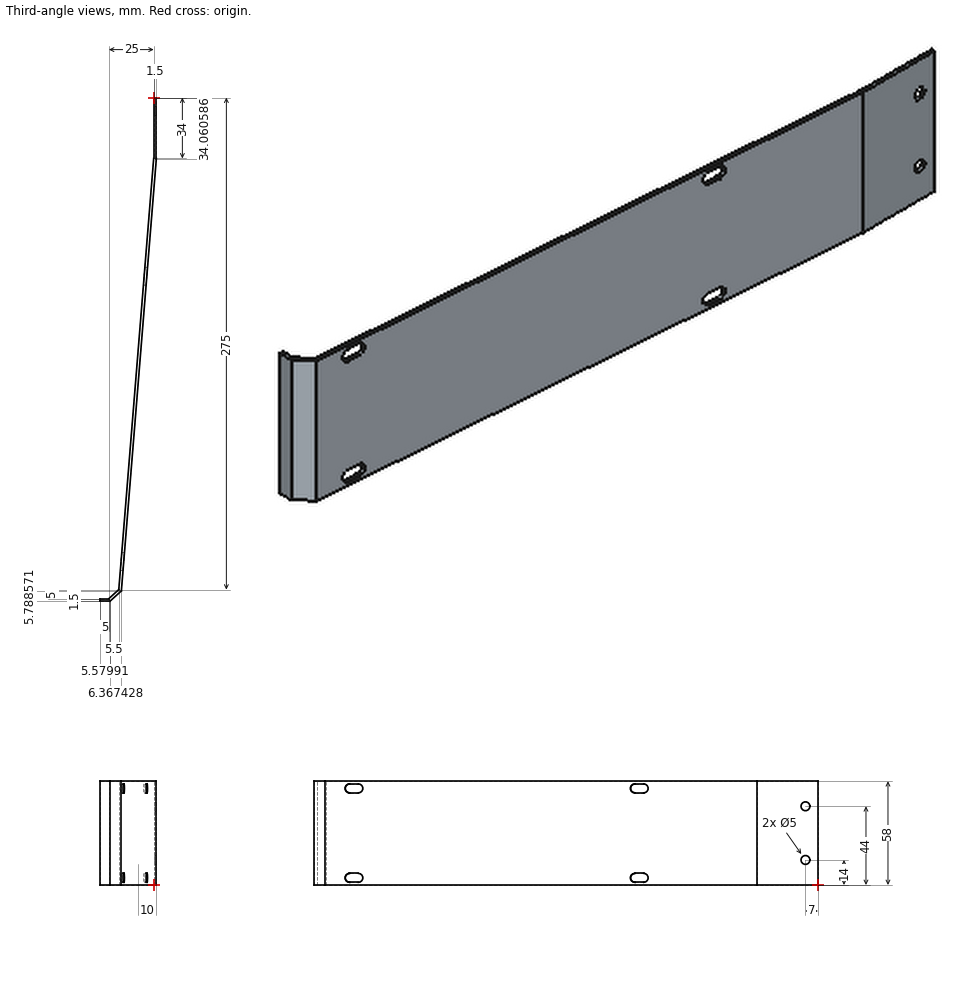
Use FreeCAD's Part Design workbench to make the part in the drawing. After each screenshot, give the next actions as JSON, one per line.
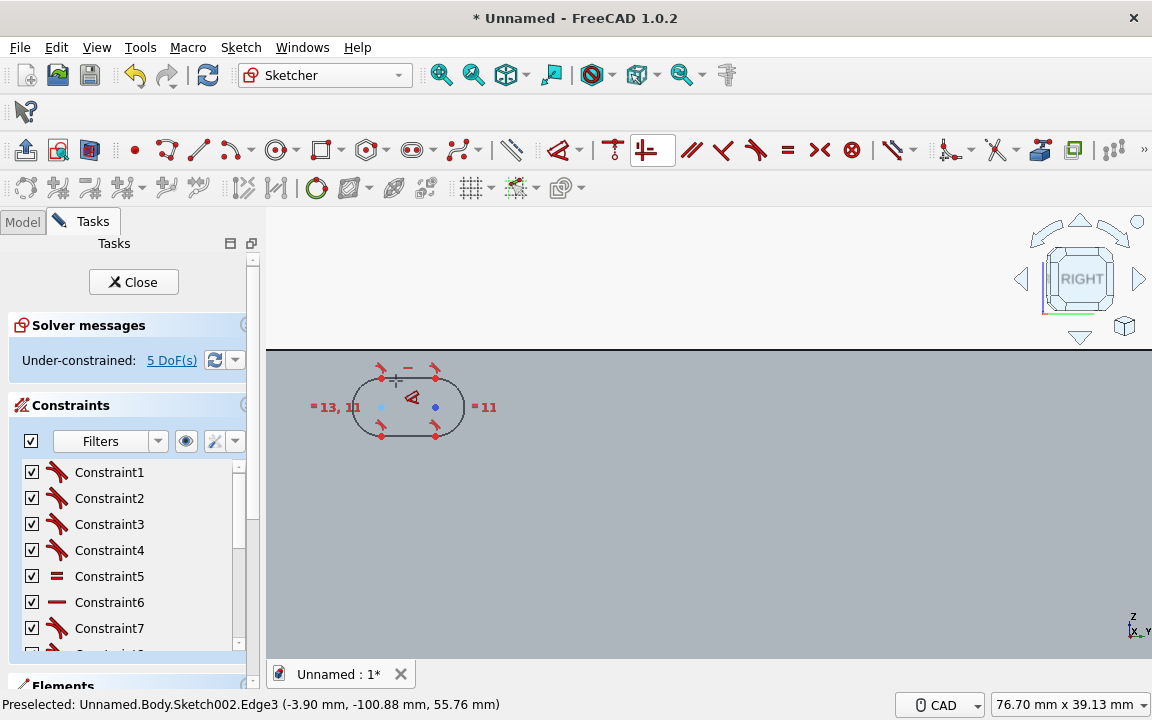
{"action": "left_click", "coordinate": [398, 378]}
{"action": "left_click", "coordinate": [408, 344]}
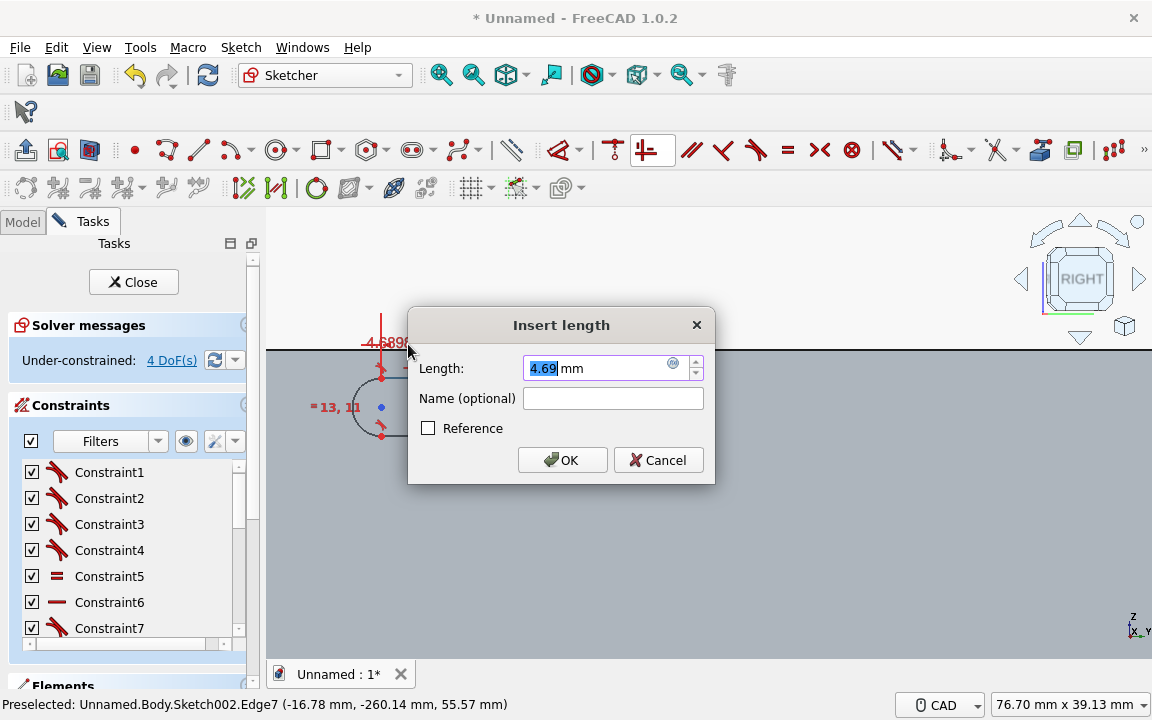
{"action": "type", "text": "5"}
{"action": "key", "text": "Return"}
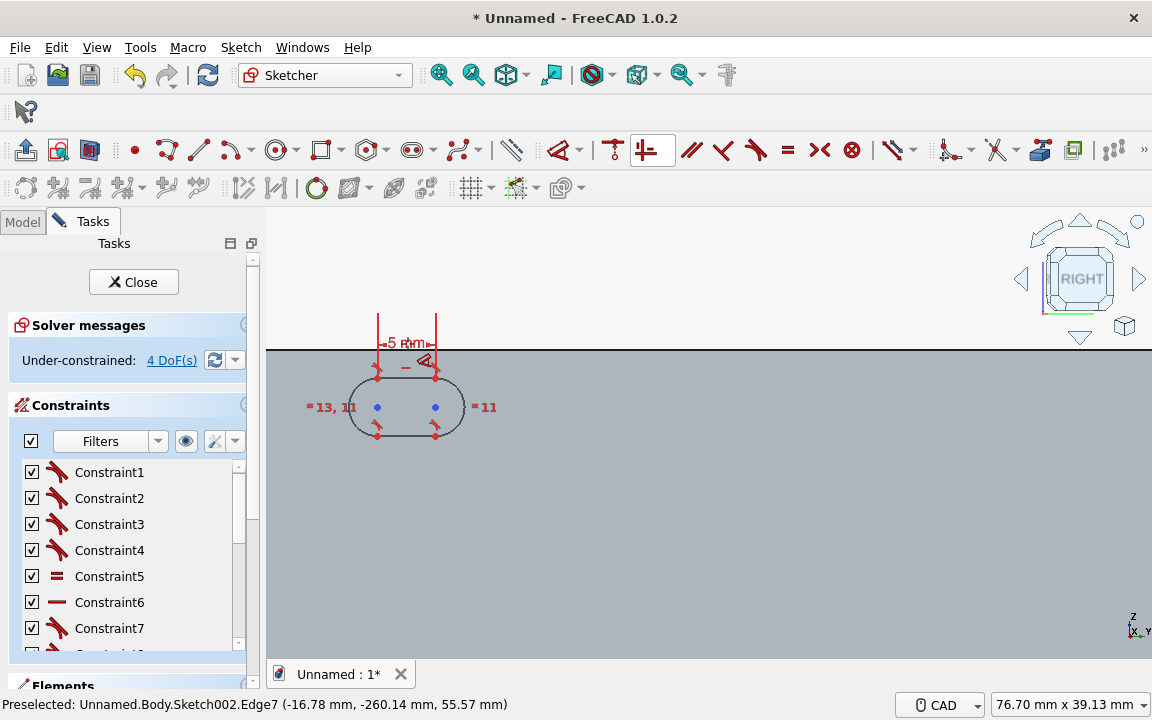
{"action": "scroll", "coordinate": [395, 381], "scroll_direction": "down", "scroll_amount": 9}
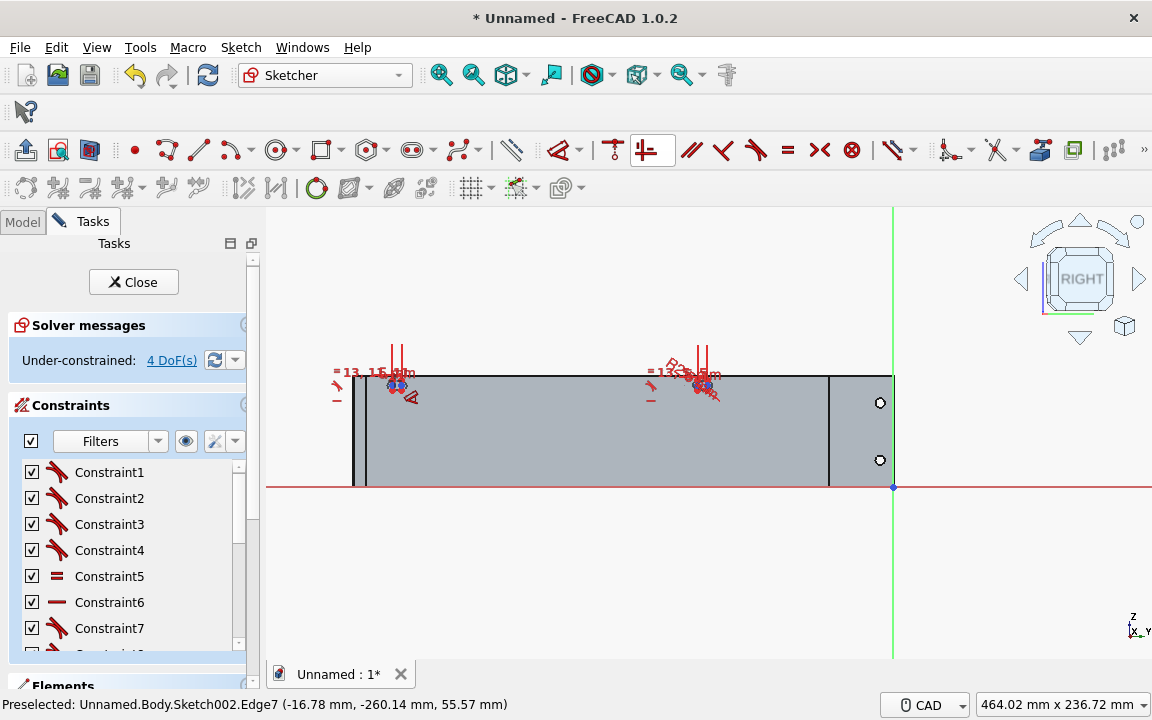
{"action": "scroll", "coordinate": [698, 385], "scroll_direction": "up", "scroll_amount": 5}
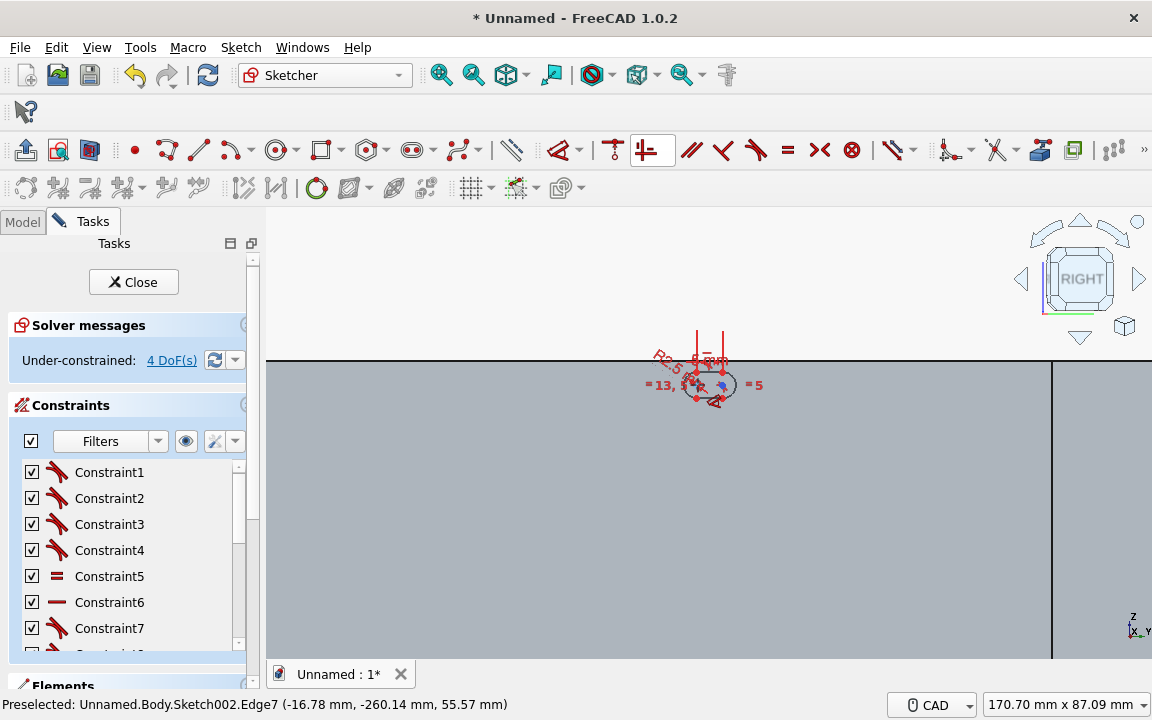
{"action": "left_click", "coordinate": [697, 385]}
{"action": "left_click", "coordinate": [663, 508]}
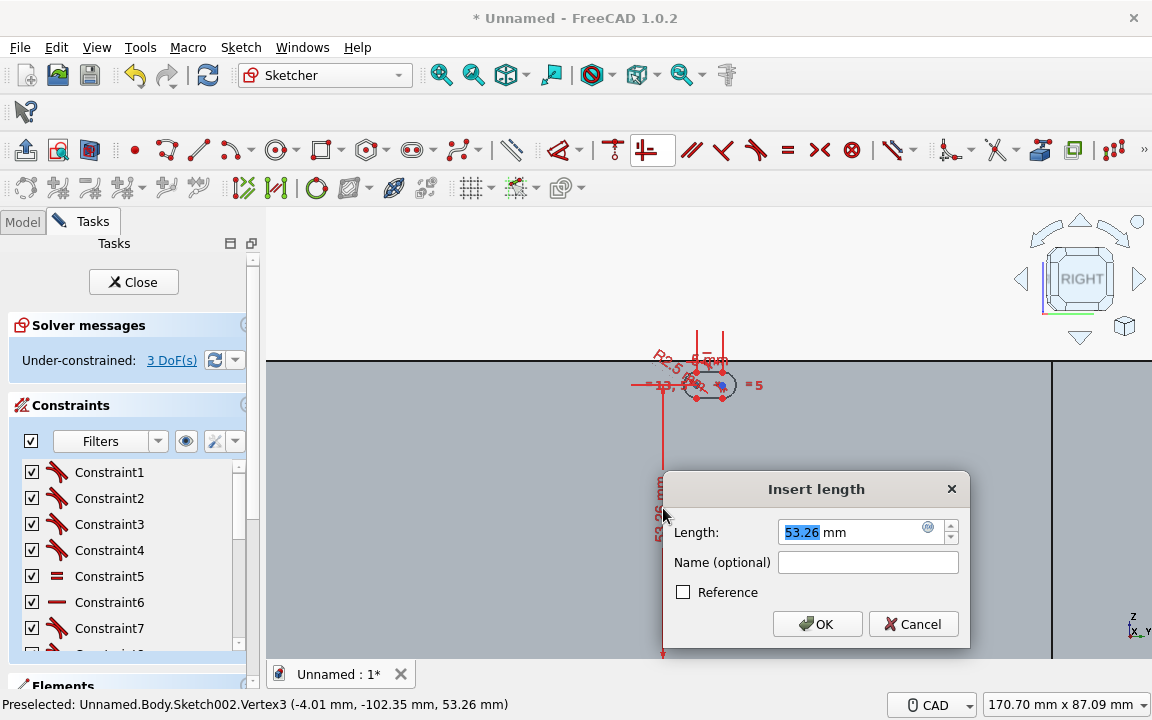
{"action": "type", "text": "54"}
{"action": "key", "text": "Return"}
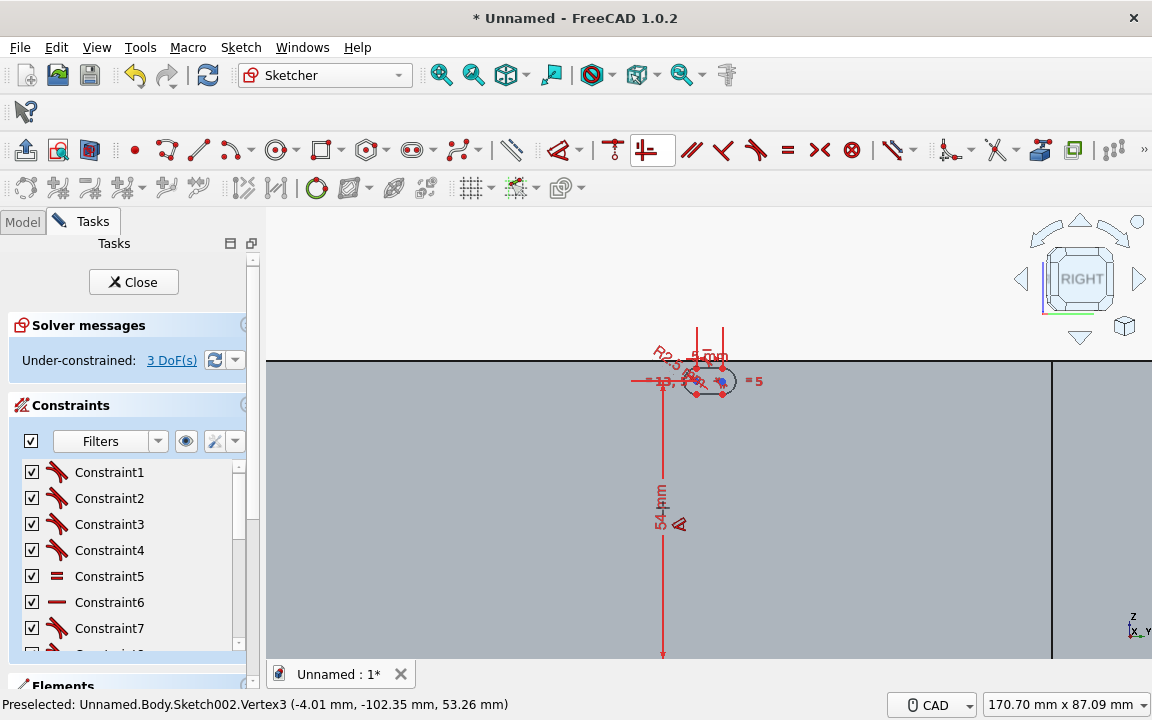
{"action": "scroll", "coordinate": [699, 385], "scroll_direction": "down", "scroll_amount": 5}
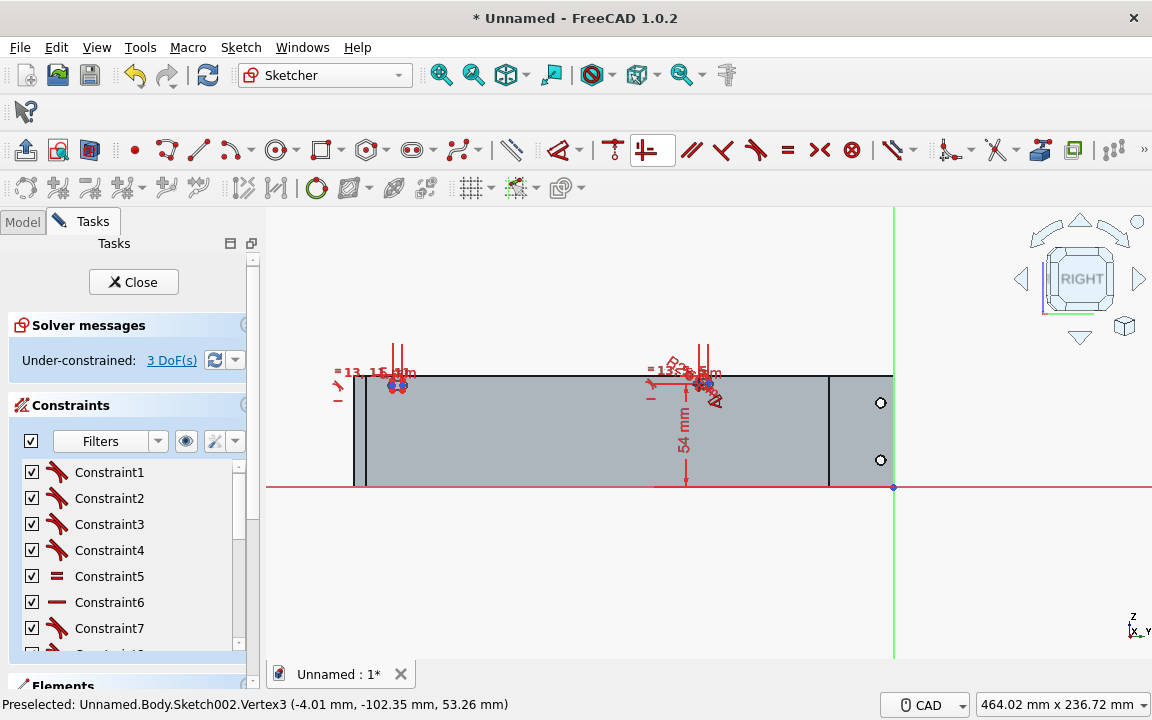
{"action": "scroll", "coordinate": [393, 386], "scroll_direction": "up", "scroll_amount": 5}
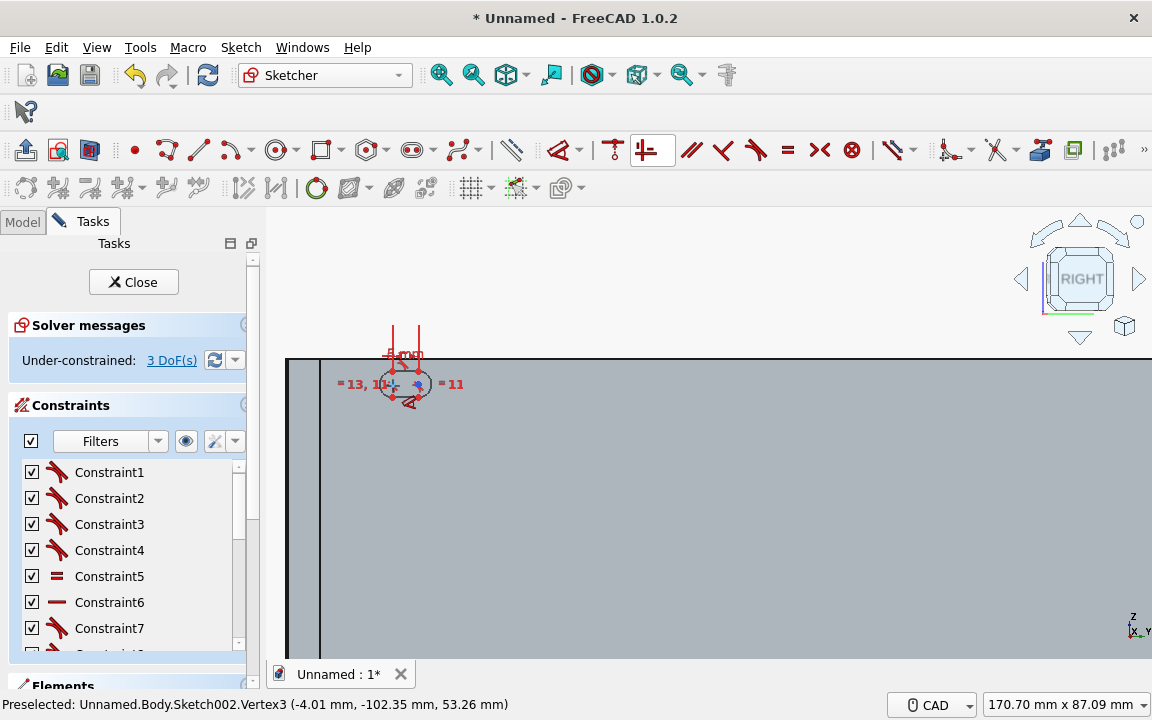
{"action": "left_click", "coordinate": [393, 384]}
{"action": "left_click", "coordinate": [359, 508]}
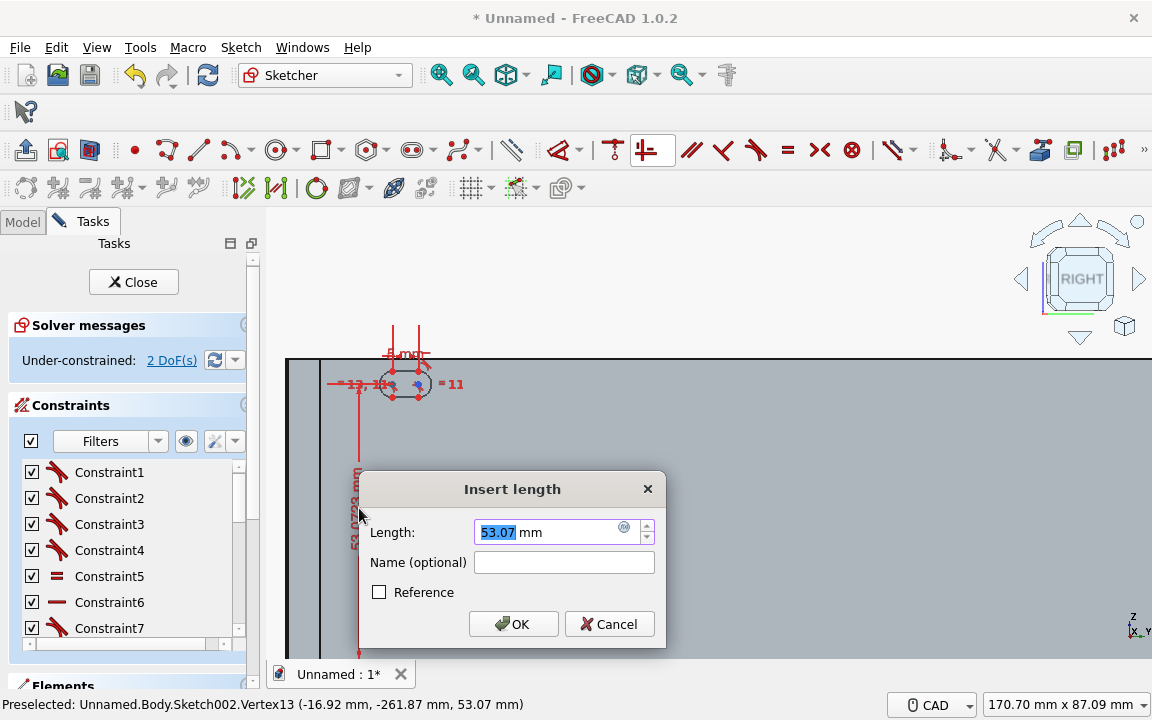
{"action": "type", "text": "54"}
{"action": "key", "text": "Return"}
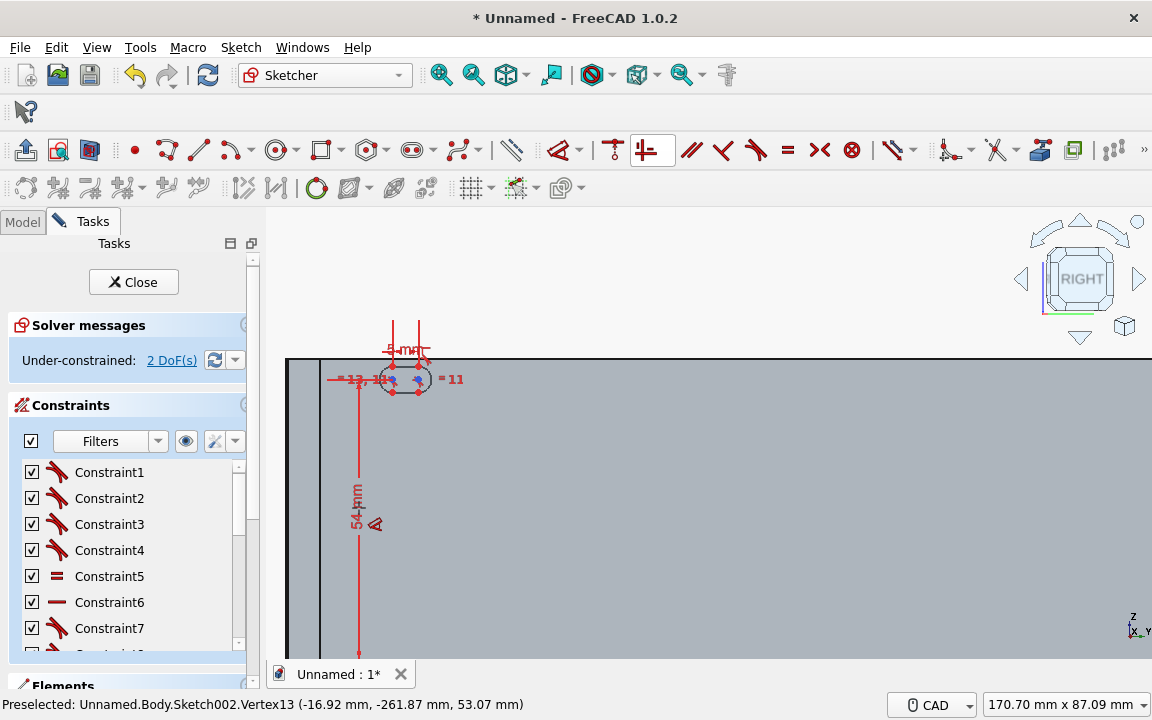
{"action": "scroll", "coordinate": [392, 386], "scroll_direction": "down", "scroll_amount": 5}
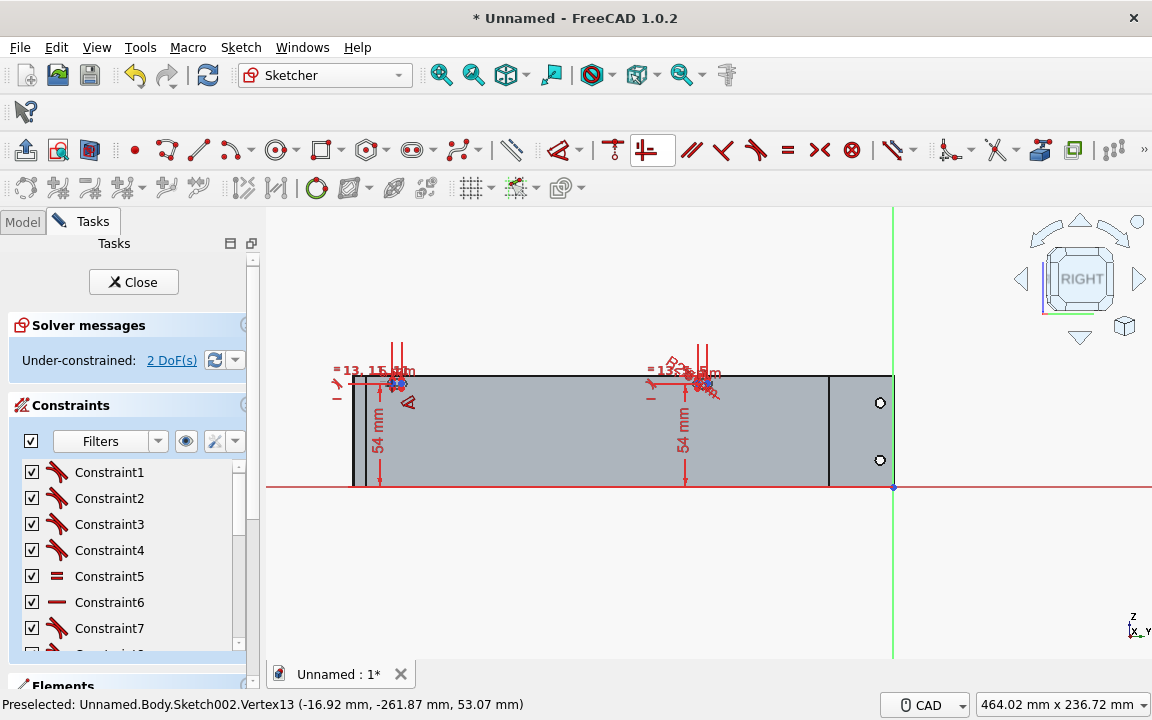
{"action": "scroll", "coordinate": [707, 389], "scroll_direction": "up", "scroll_amount": 5}